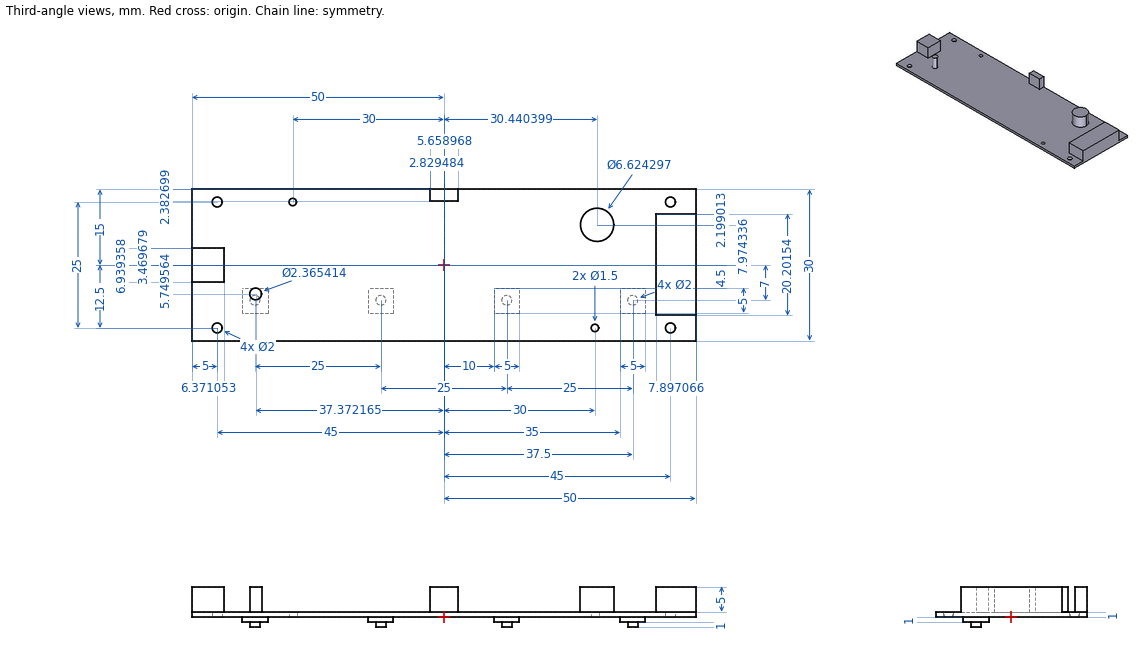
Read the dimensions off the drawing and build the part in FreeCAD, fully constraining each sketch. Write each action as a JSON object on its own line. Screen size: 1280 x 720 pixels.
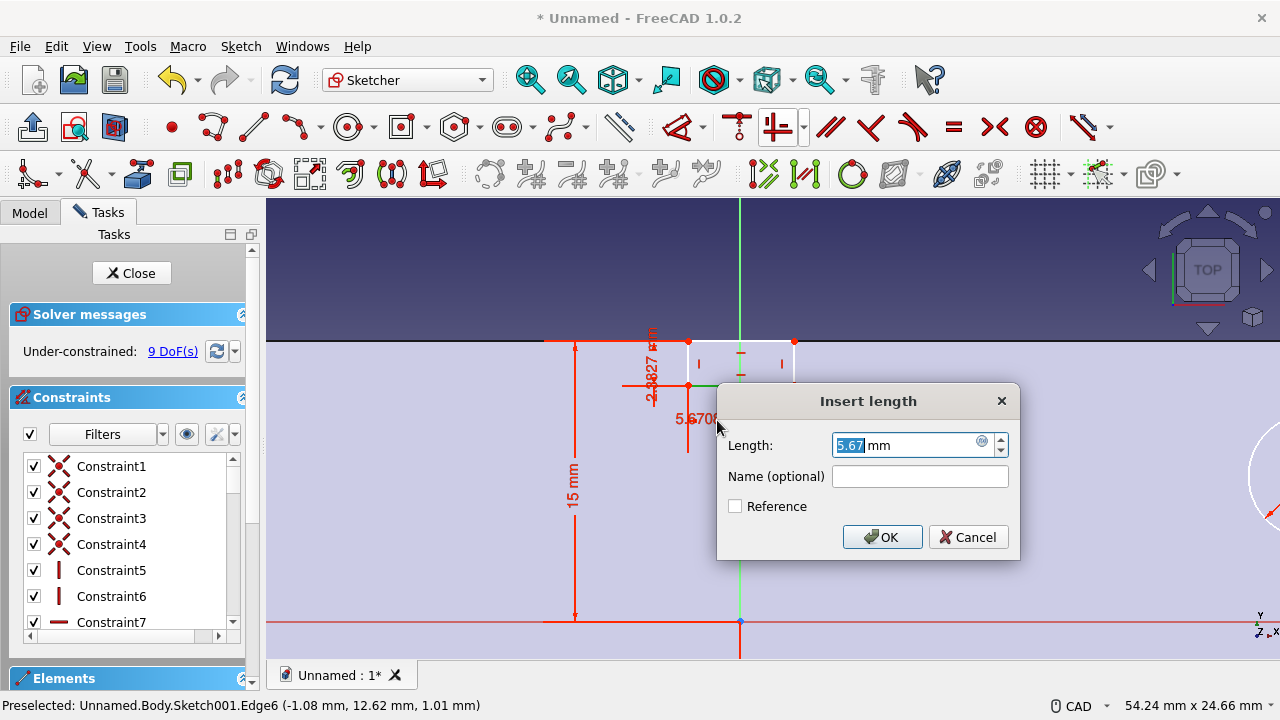
{"action": "type", "text": "5.658968"}
{"action": "key", "text": "Return"}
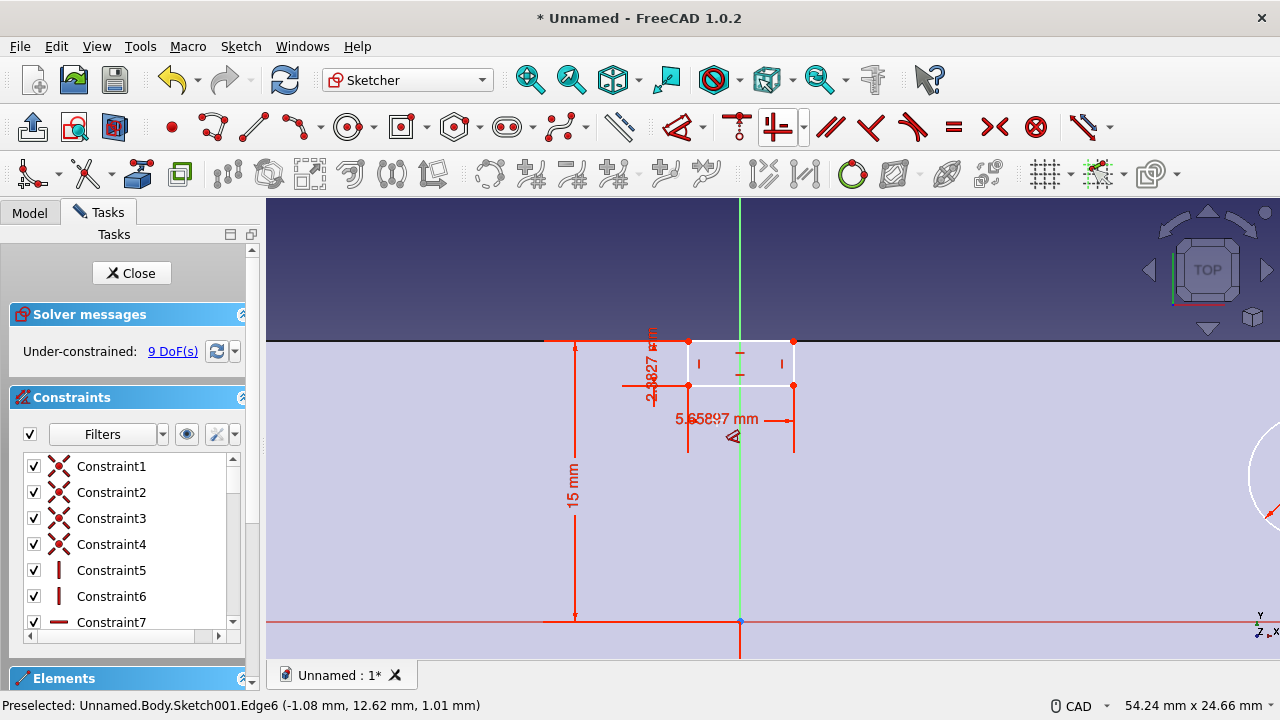
{"action": "scroll", "coordinate": [689, 365], "scroll_direction": "down", "scroll_amount": 6}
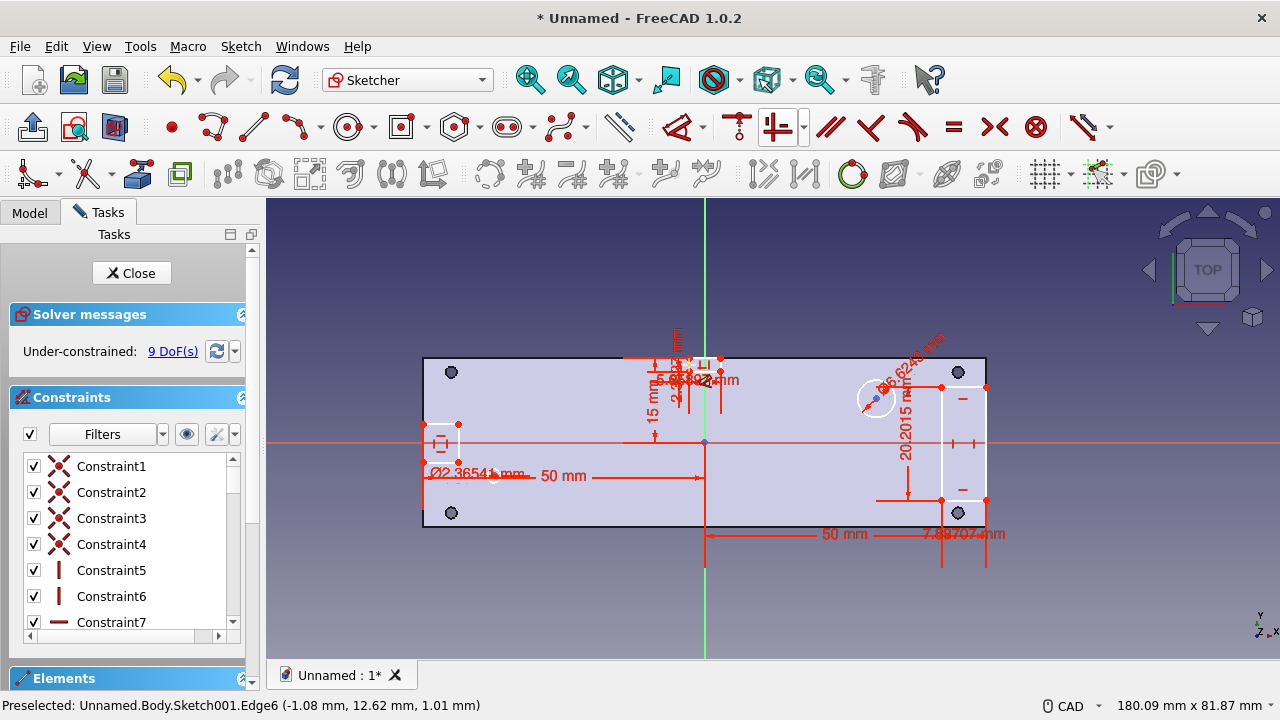
{"action": "scroll", "coordinate": [423, 436], "scroll_direction": "up", "scroll_amount": 4}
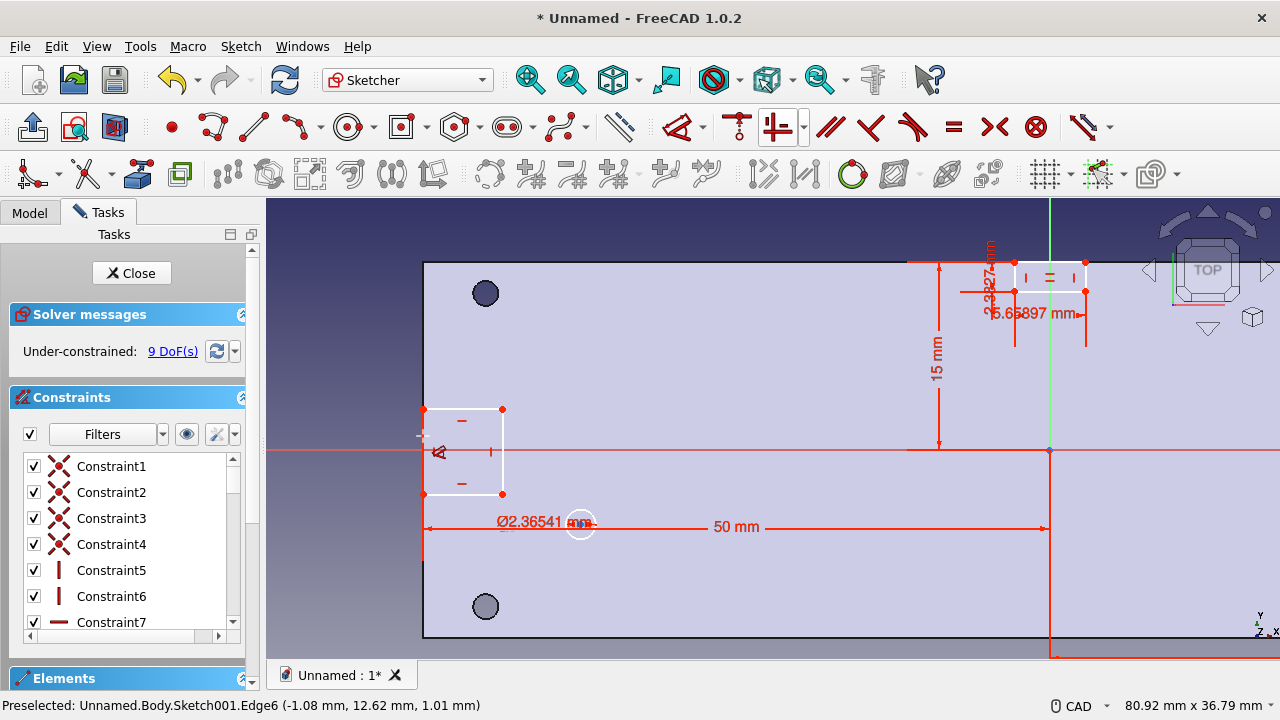
{"action": "left_click", "coordinate": [423, 435]}
{"action": "left_click", "coordinate": [389, 432]}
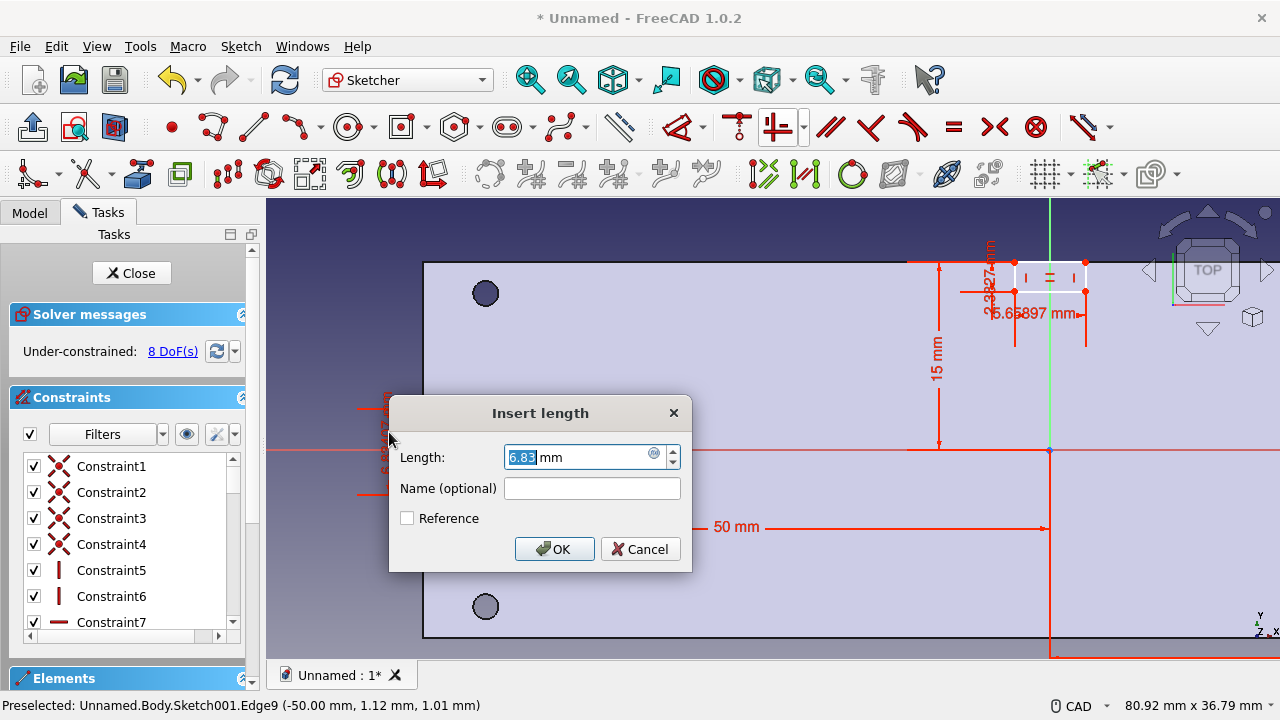
{"action": "type", "text": "6.939358"}
{"action": "key", "text": "Return"}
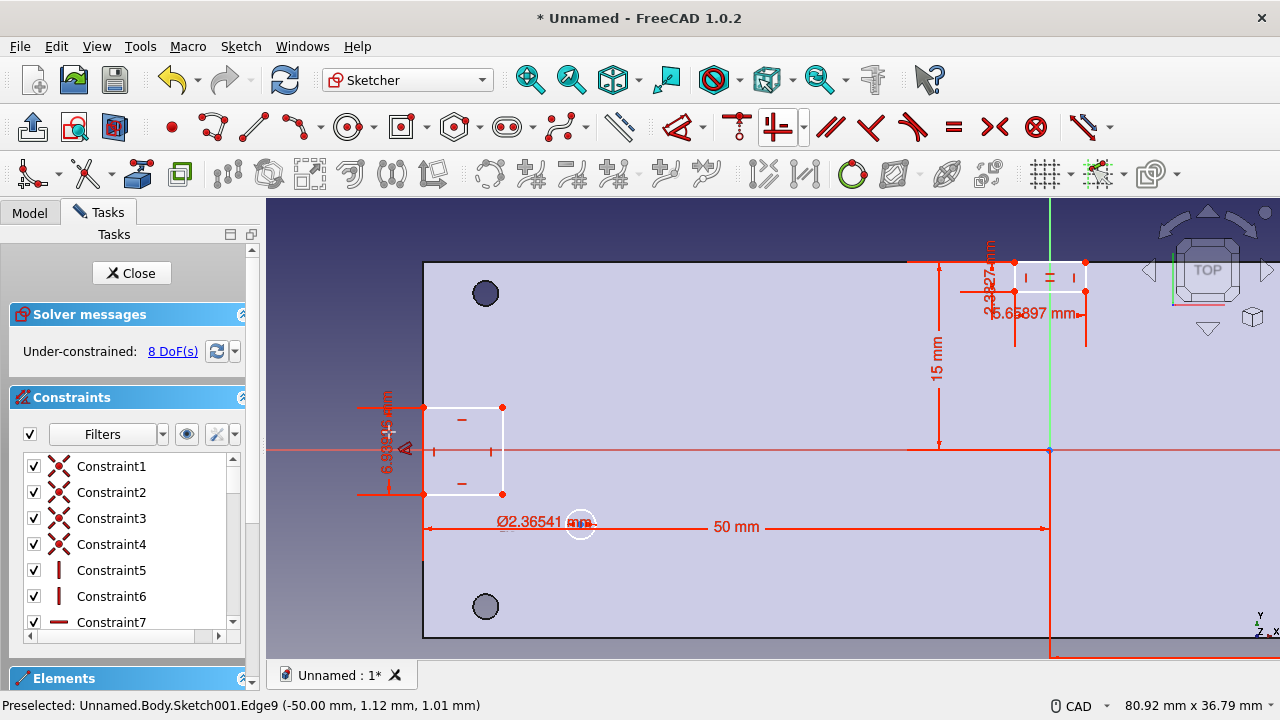
{"action": "left_click", "coordinate": [447, 495]}
{"action": "left_click", "coordinate": [463, 529]}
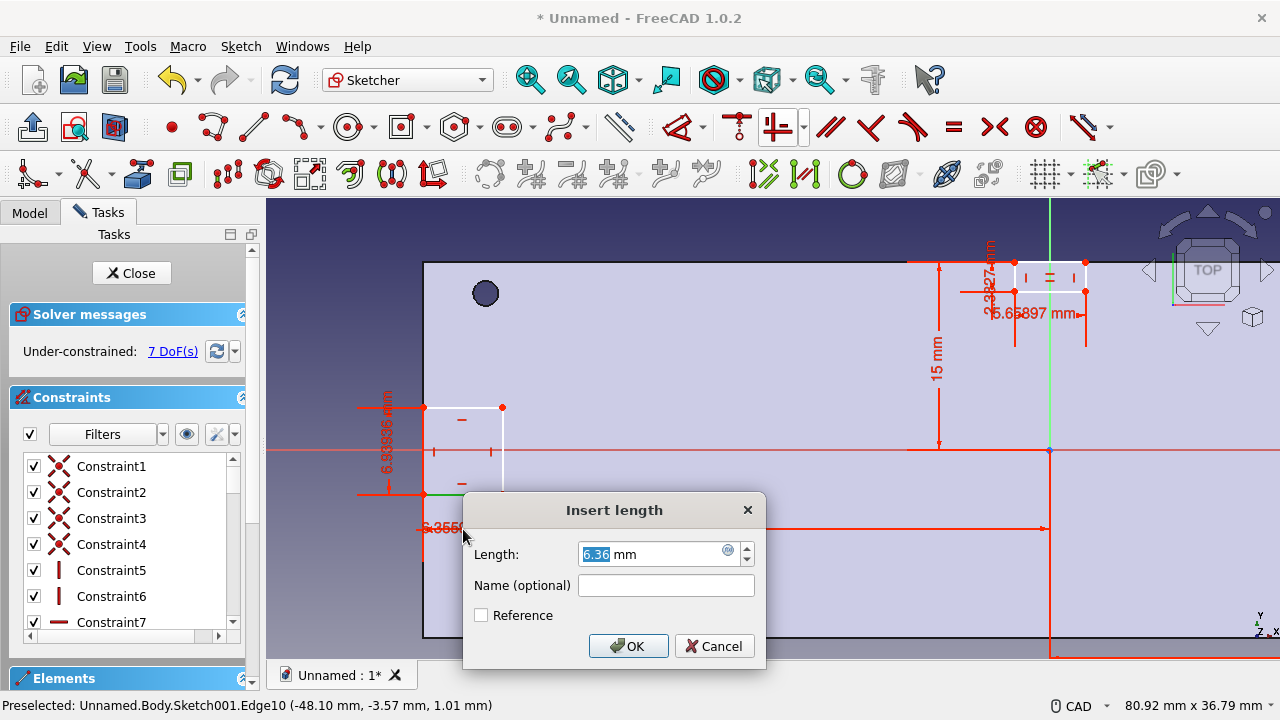
{"action": "type", "text": "6.371053"}
{"action": "key", "text": "Return"}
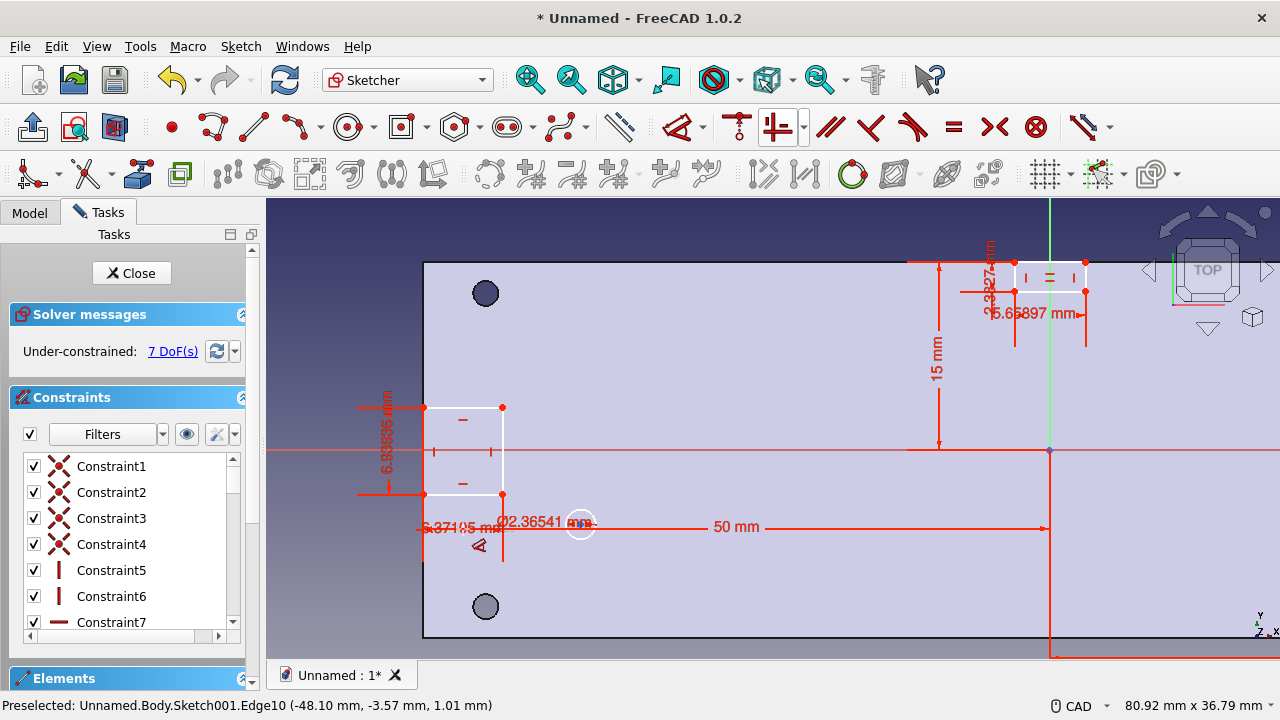
{"action": "scroll", "coordinate": [423, 436], "scroll_direction": "down", "scroll_amount": 4}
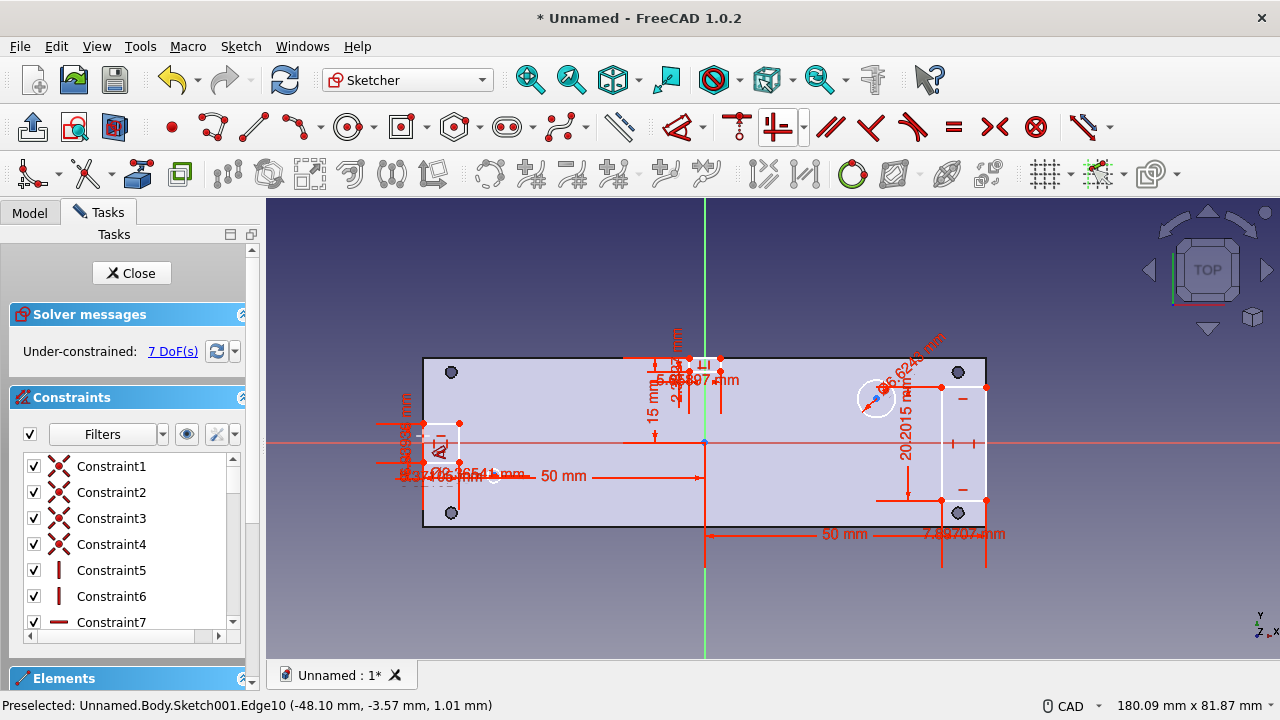
{"action": "left_click", "coordinate": [876, 399]}
{"action": "left_click", "coordinate": [671, 421]}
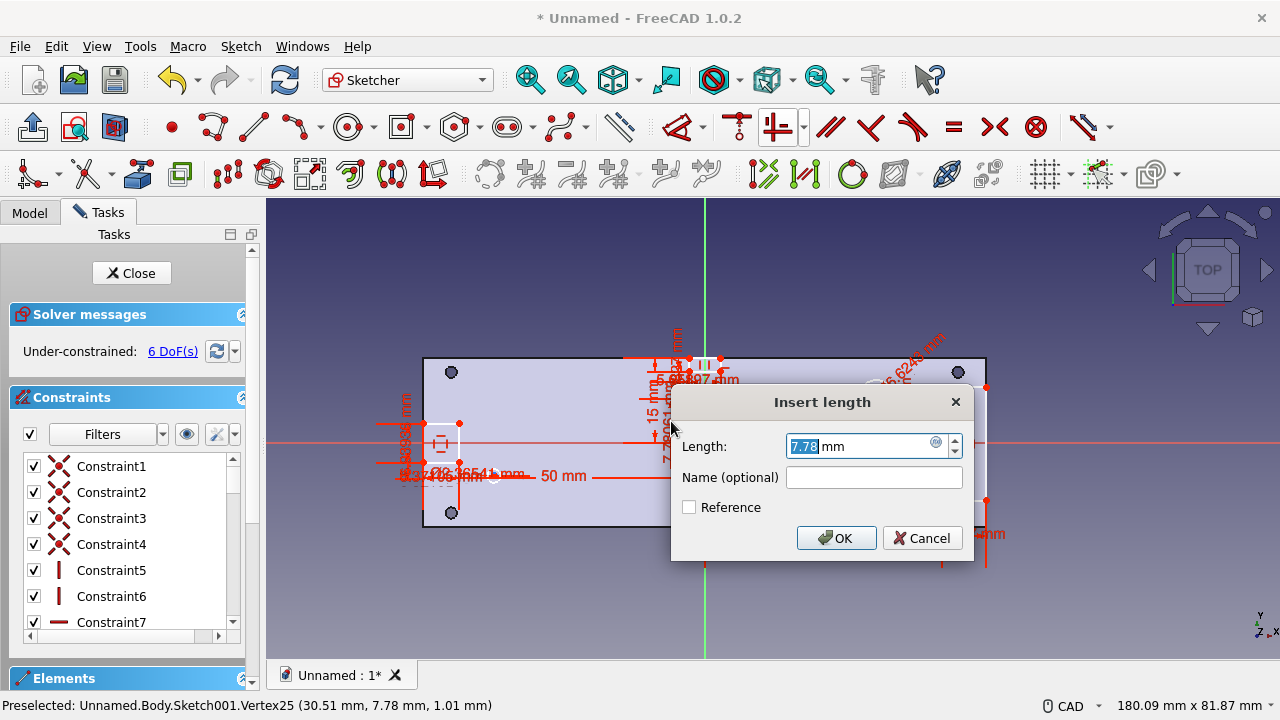
{"action": "type", "text": "7.974336"}
{"action": "key", "text": "Return"}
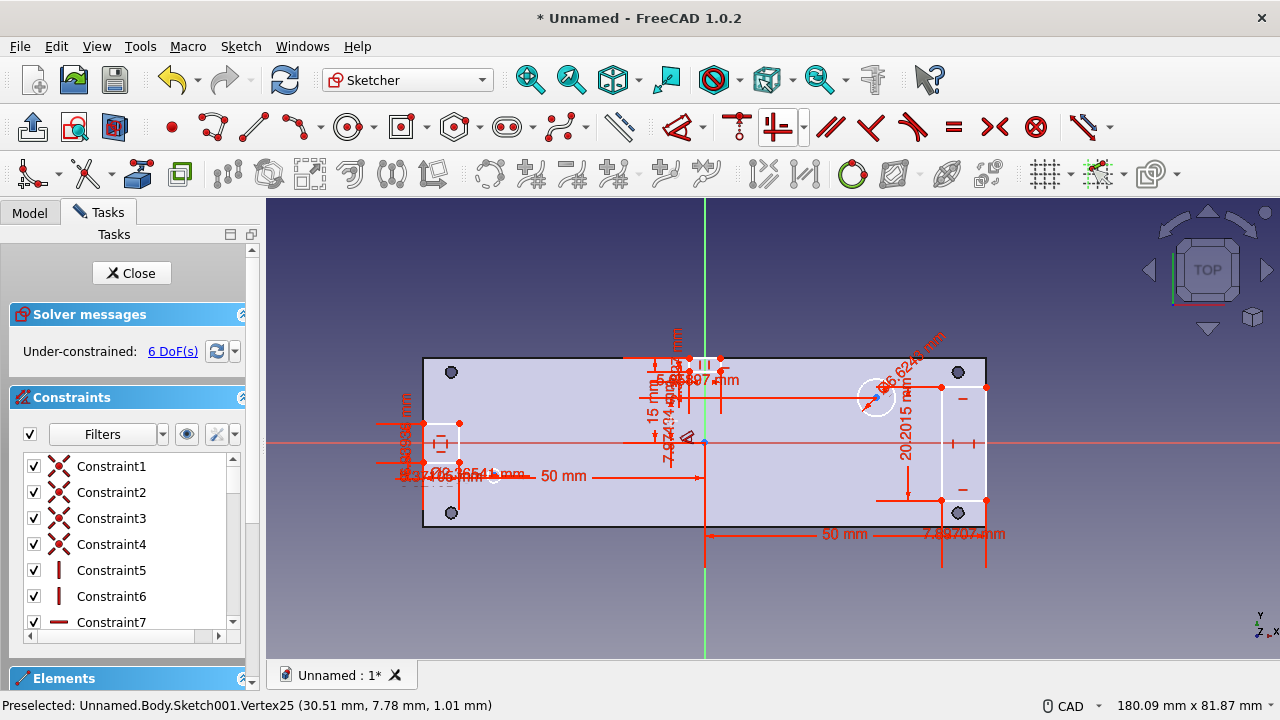
{"action": "scroll", "coordinate": [494, 476], "scroll_direction": "up", "scroll_amount": 2}